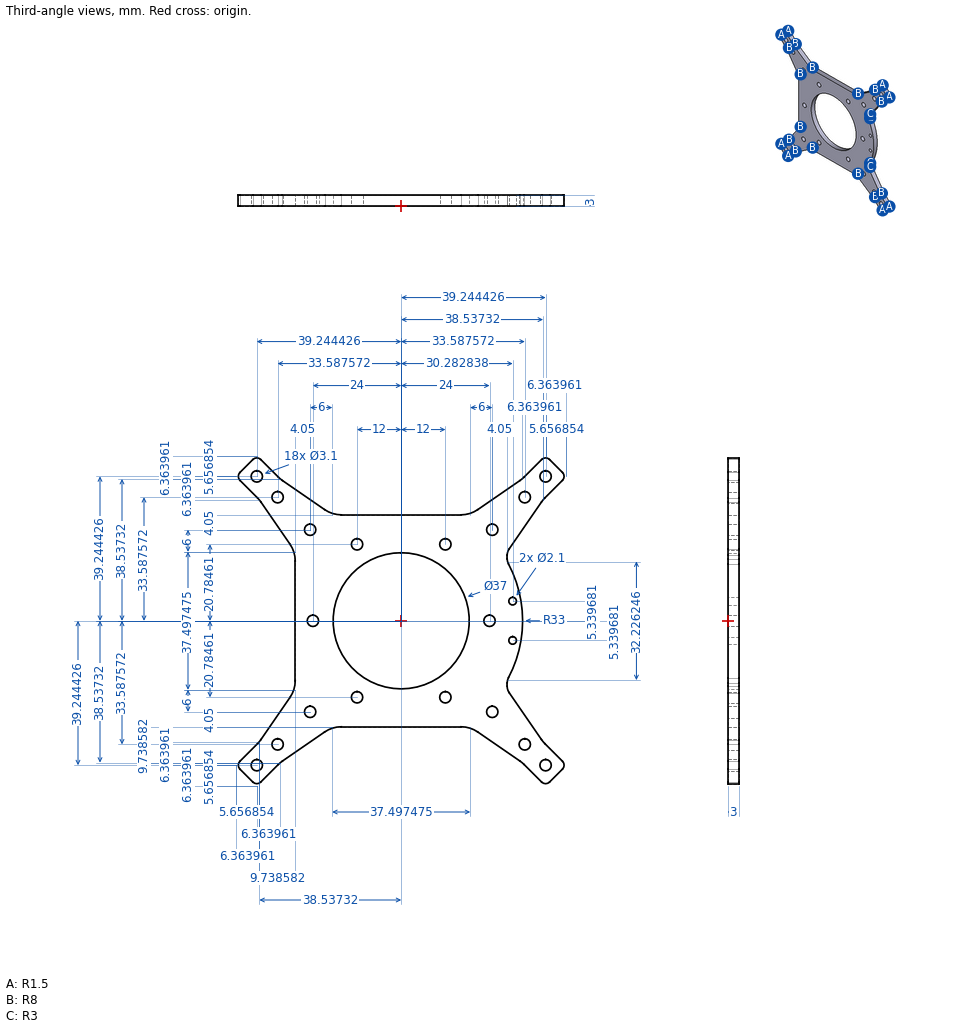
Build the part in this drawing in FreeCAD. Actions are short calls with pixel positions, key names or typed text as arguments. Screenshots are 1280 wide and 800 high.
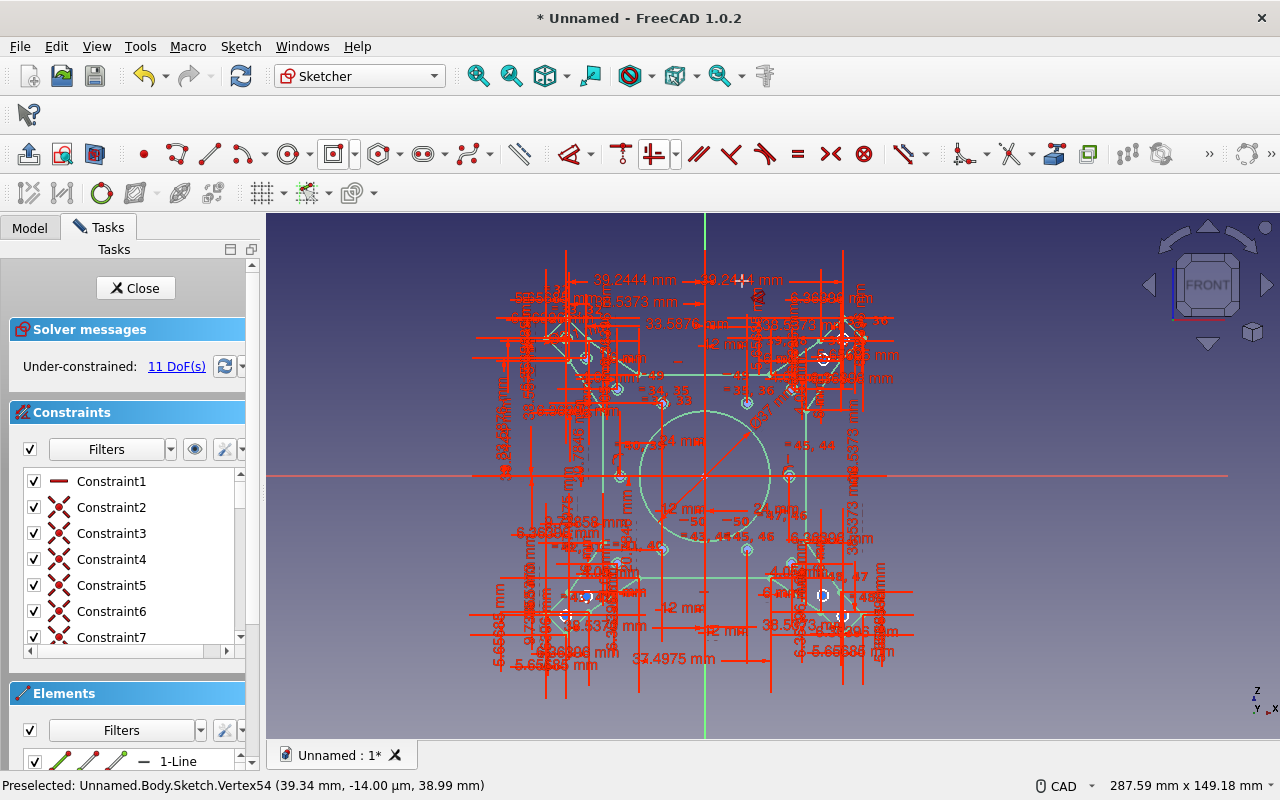
click(843, 339)
click(901, 408)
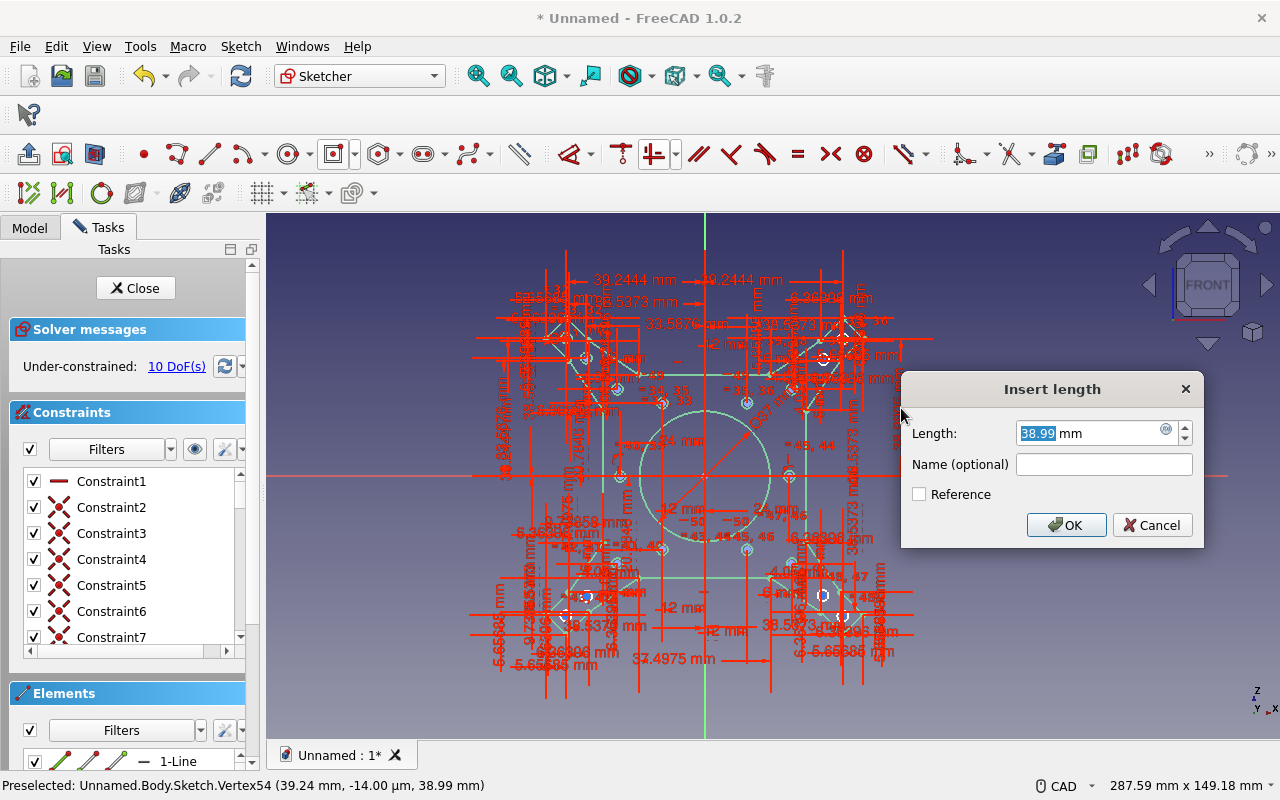
text(39.244426)
key(Return)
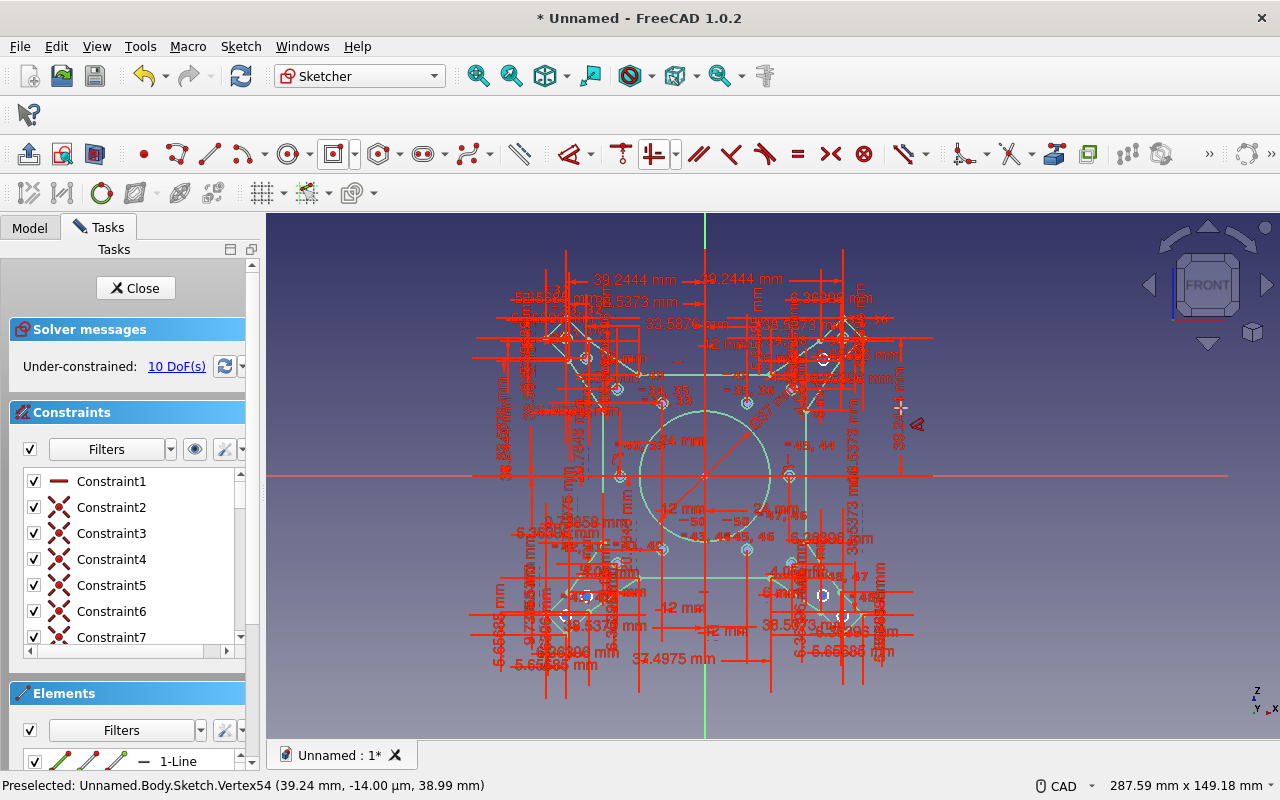
click(824, 359)
click(737, 301)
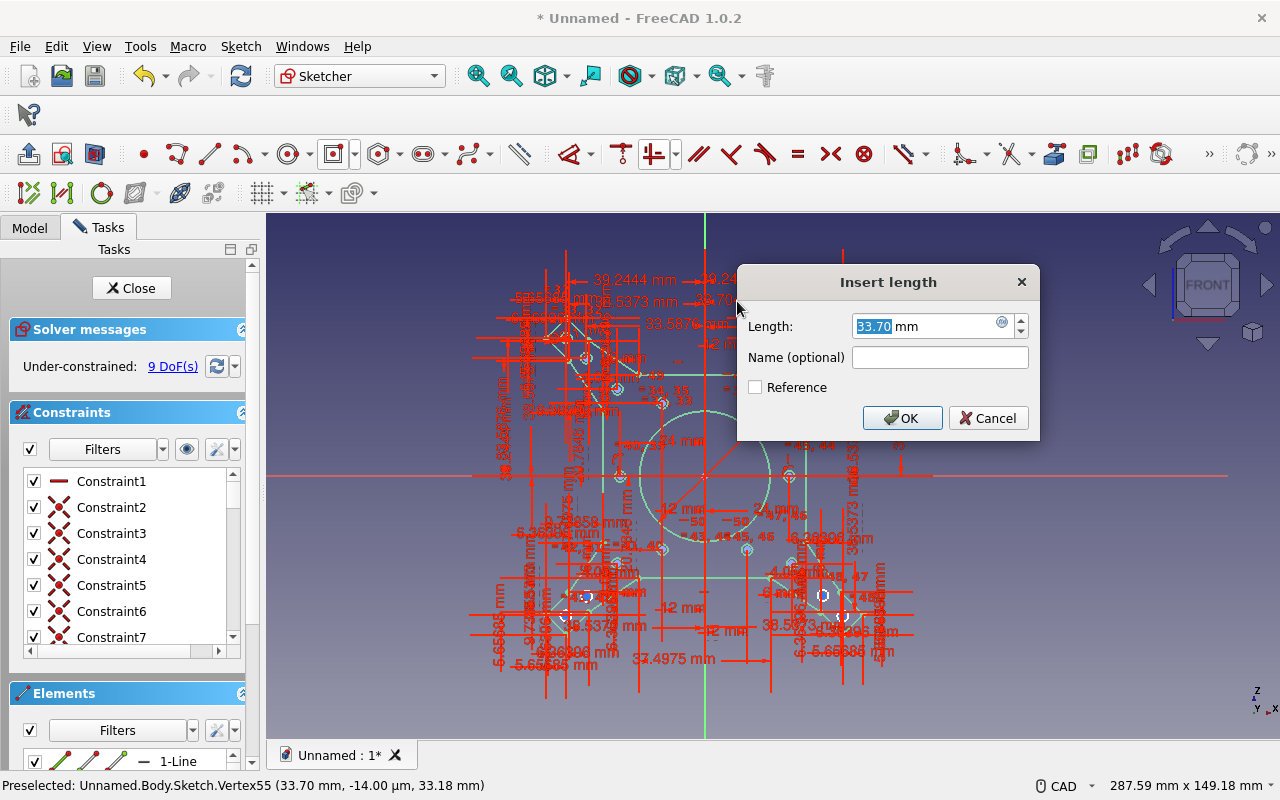
text(33.587572)
key(Return)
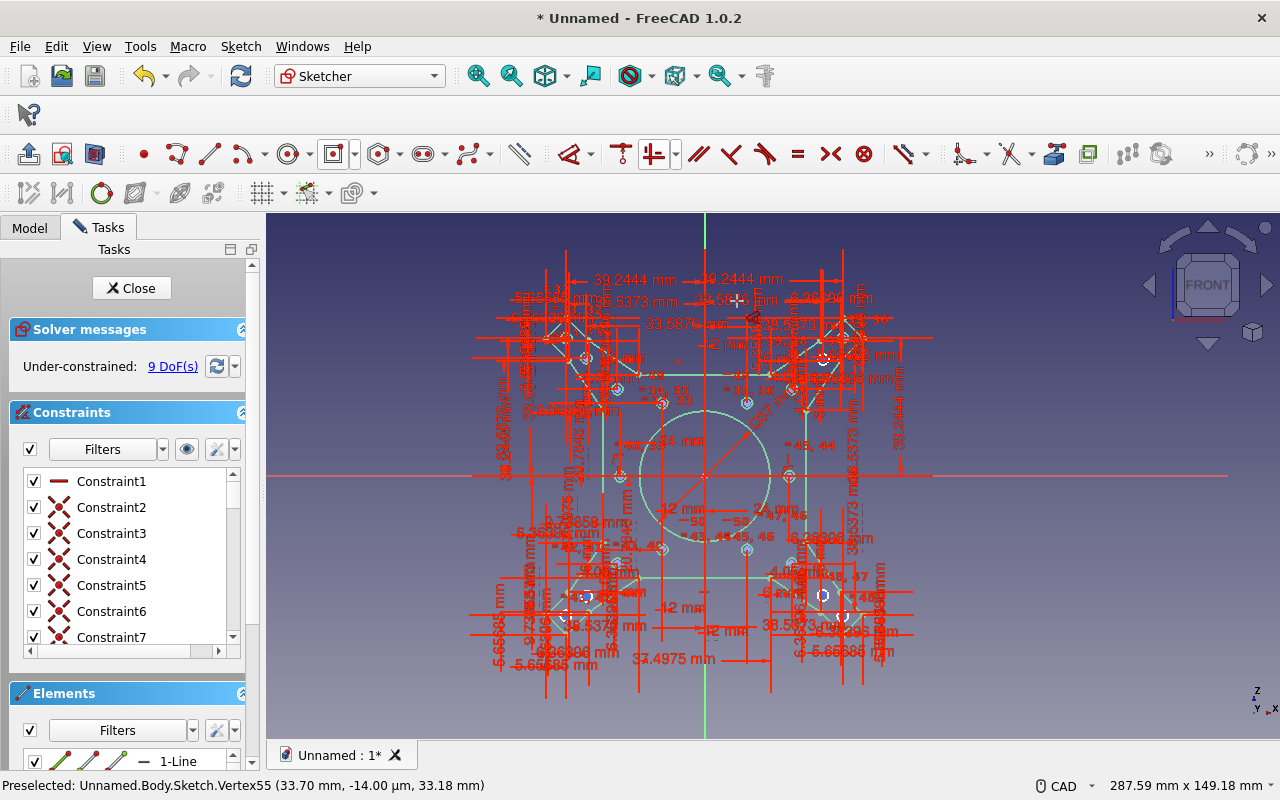
click(823, 359)
click(929, 445)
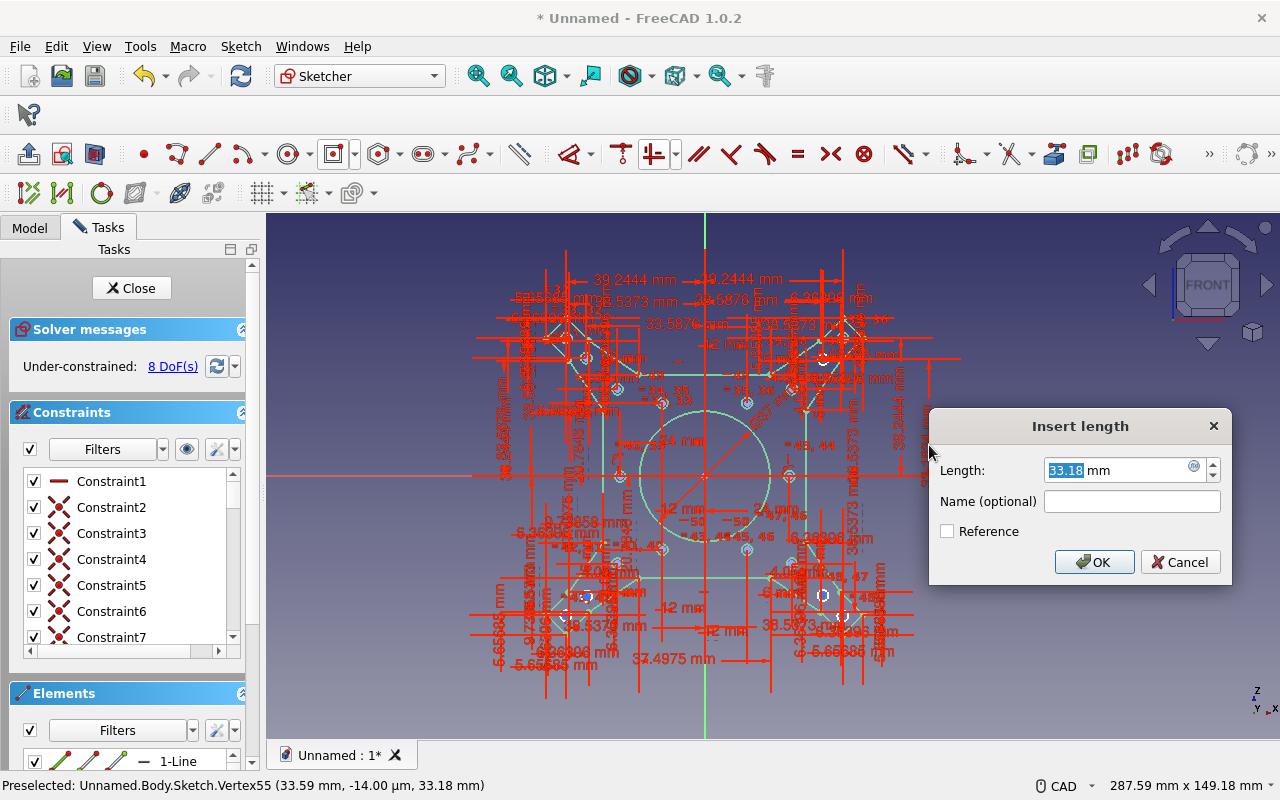
text(33.587572)
key(Return)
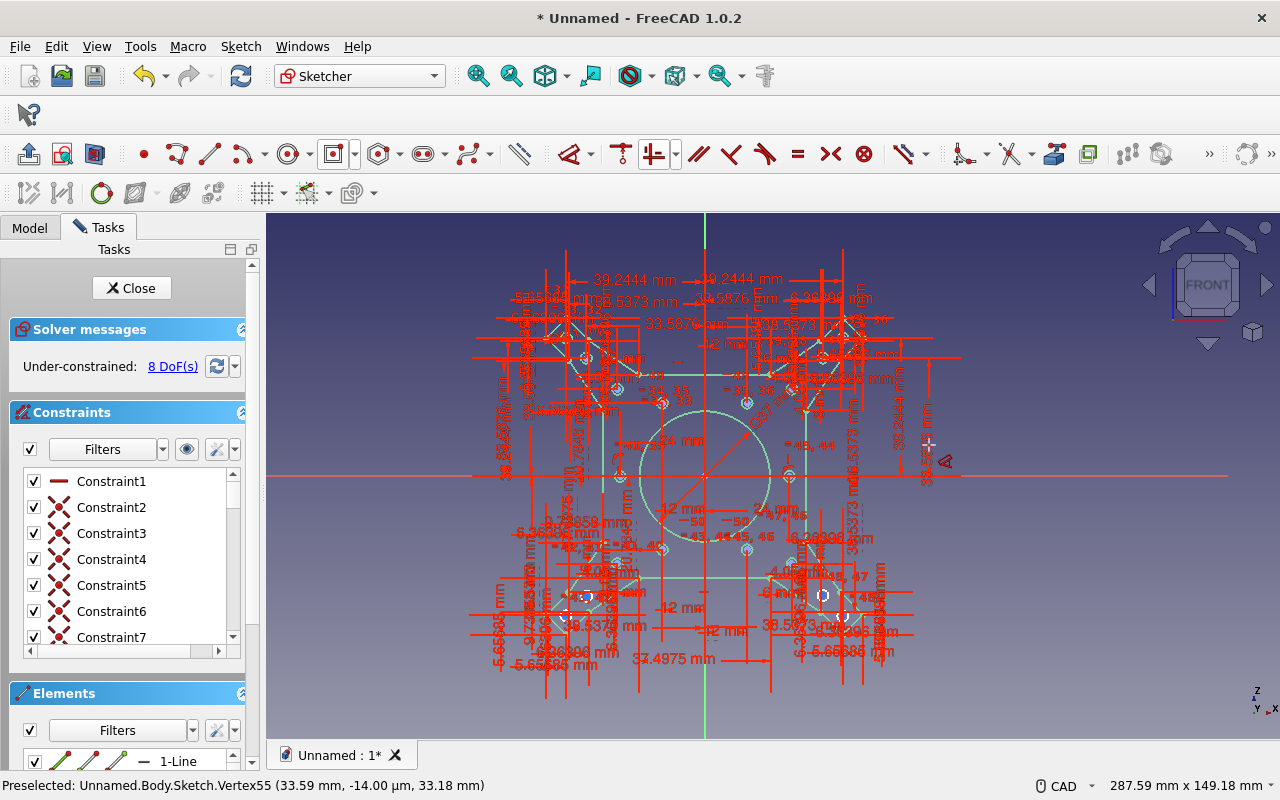
click(587, 596)
click(687, 394)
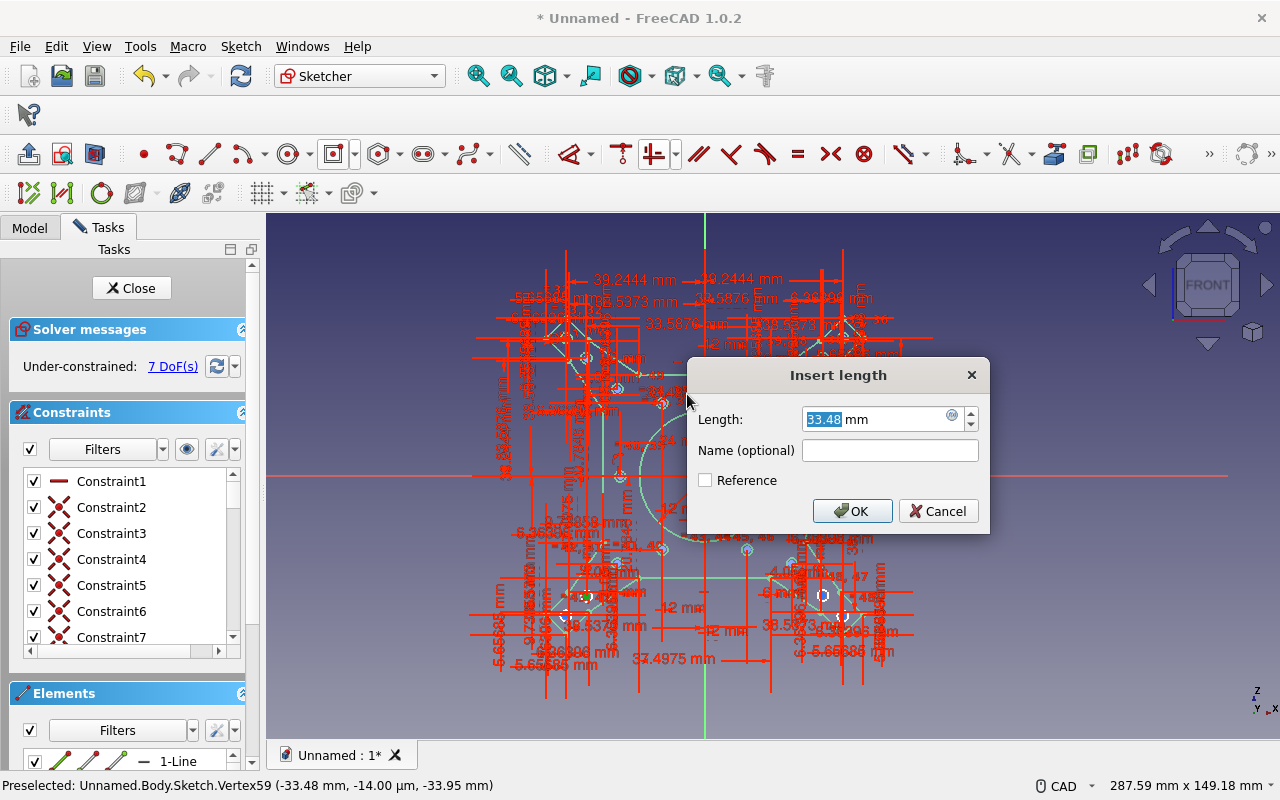
text(33.587572)
key(Return)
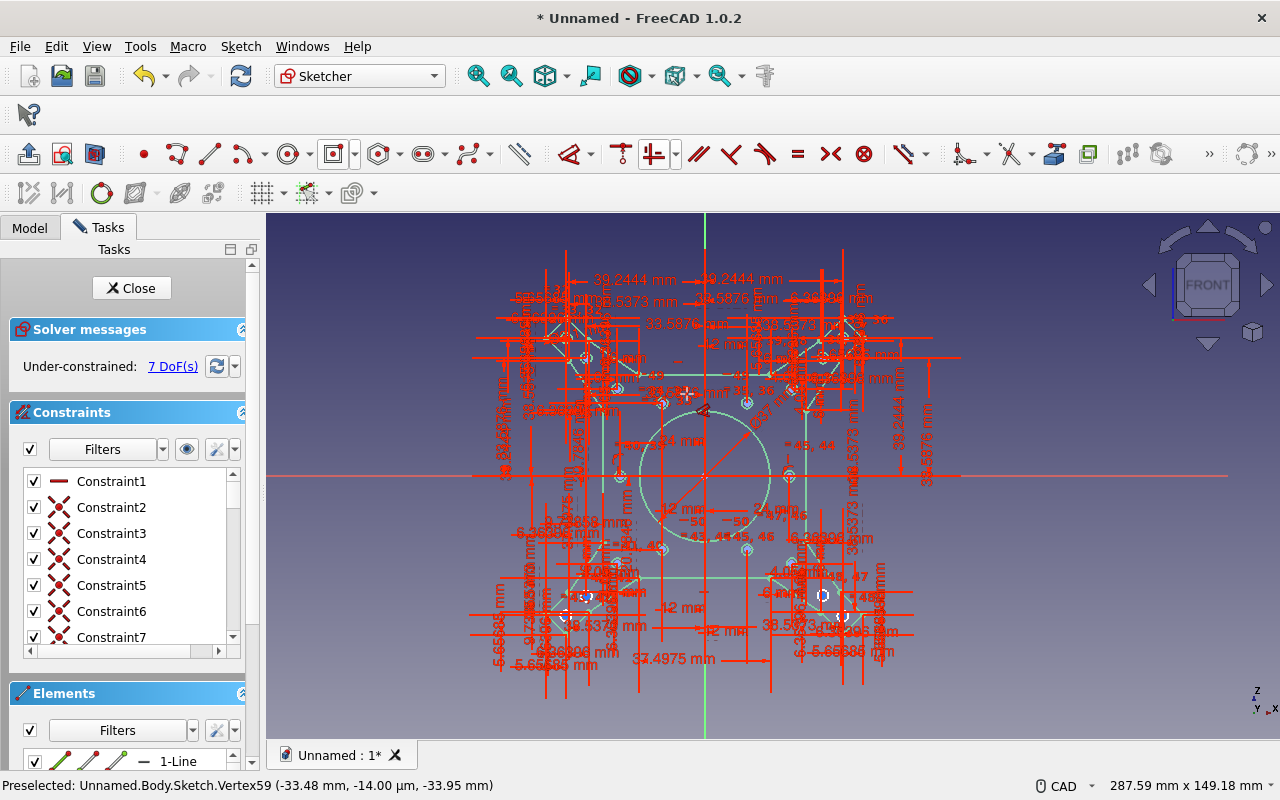
click(586, 596)
click(480, 536)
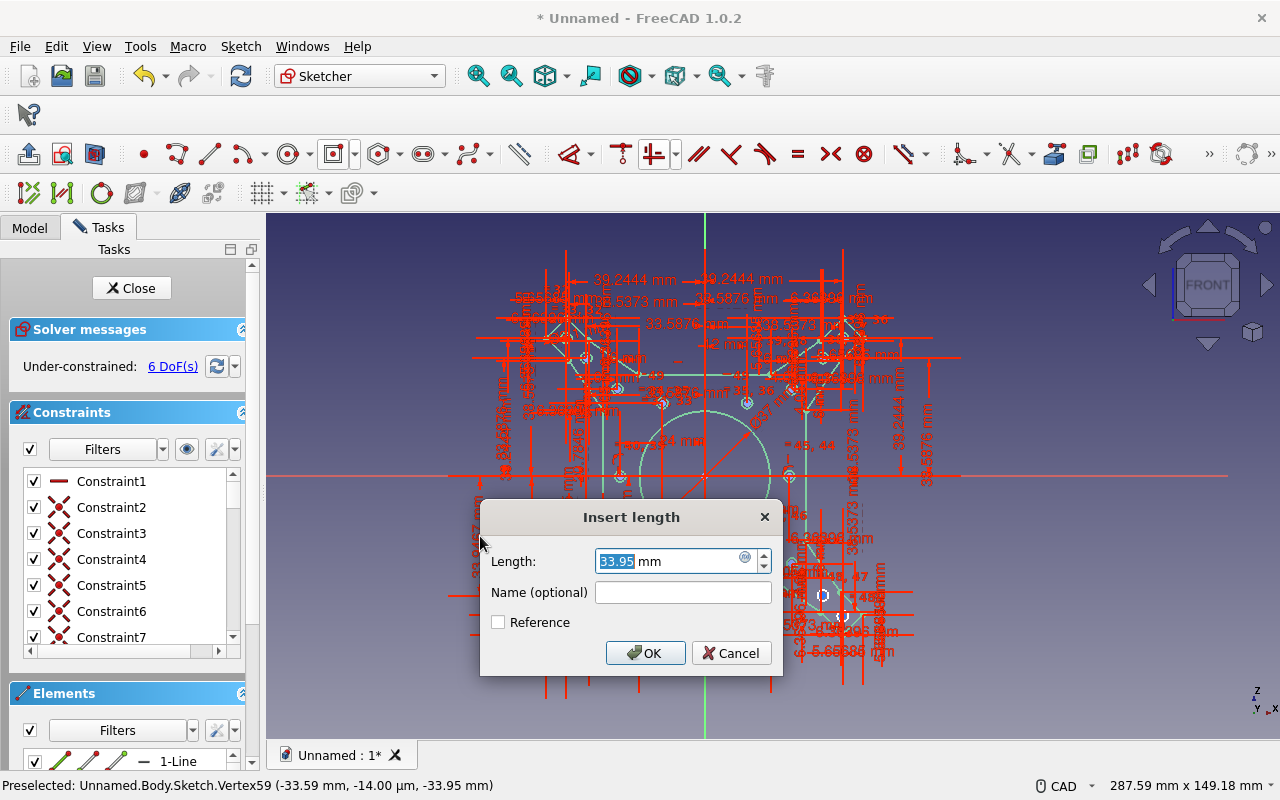
text(33.587572)
key(Return)